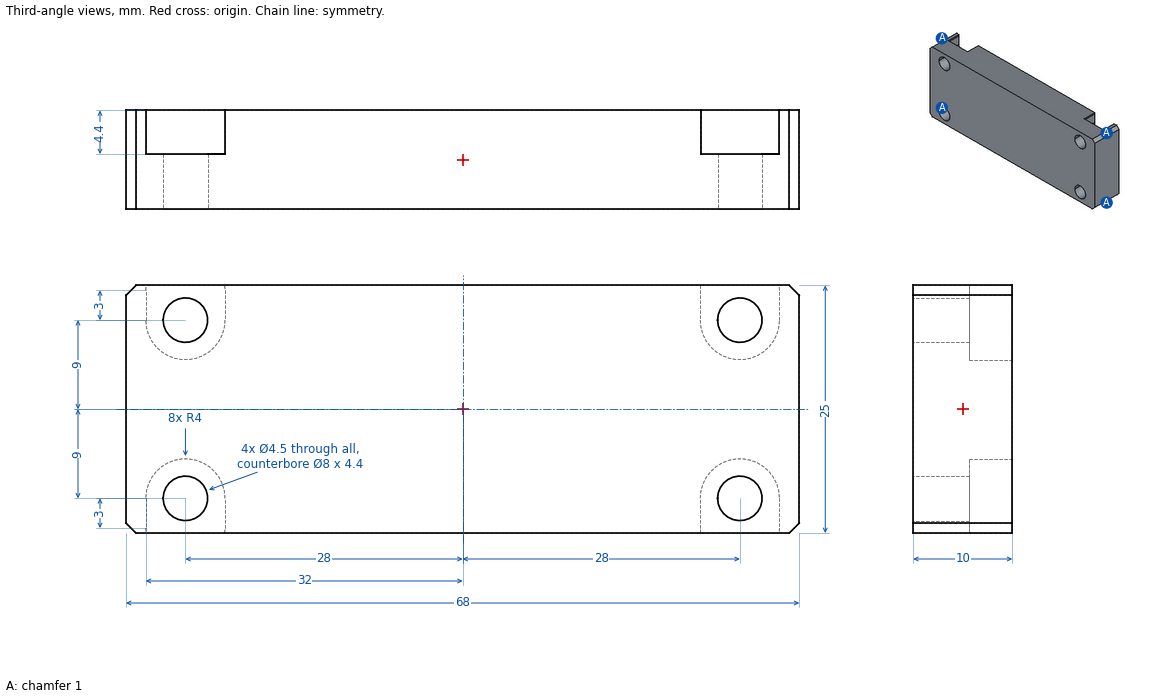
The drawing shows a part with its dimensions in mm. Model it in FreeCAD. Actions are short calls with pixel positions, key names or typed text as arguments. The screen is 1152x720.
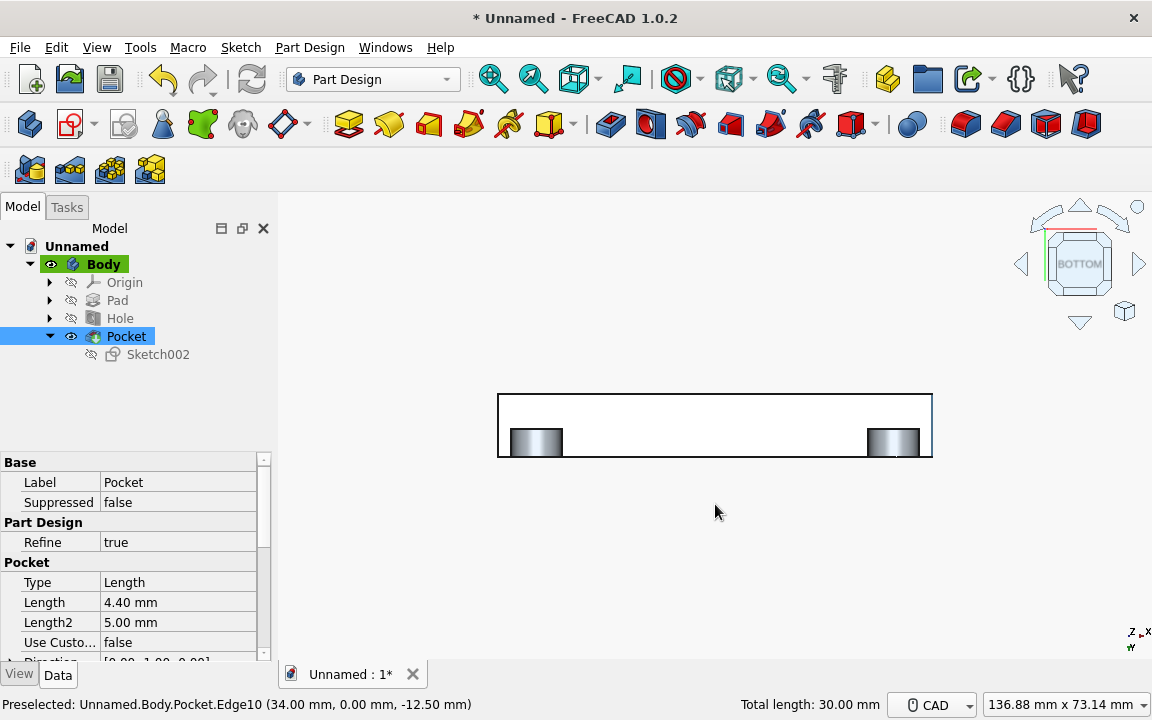
click(498, 424, ctrl)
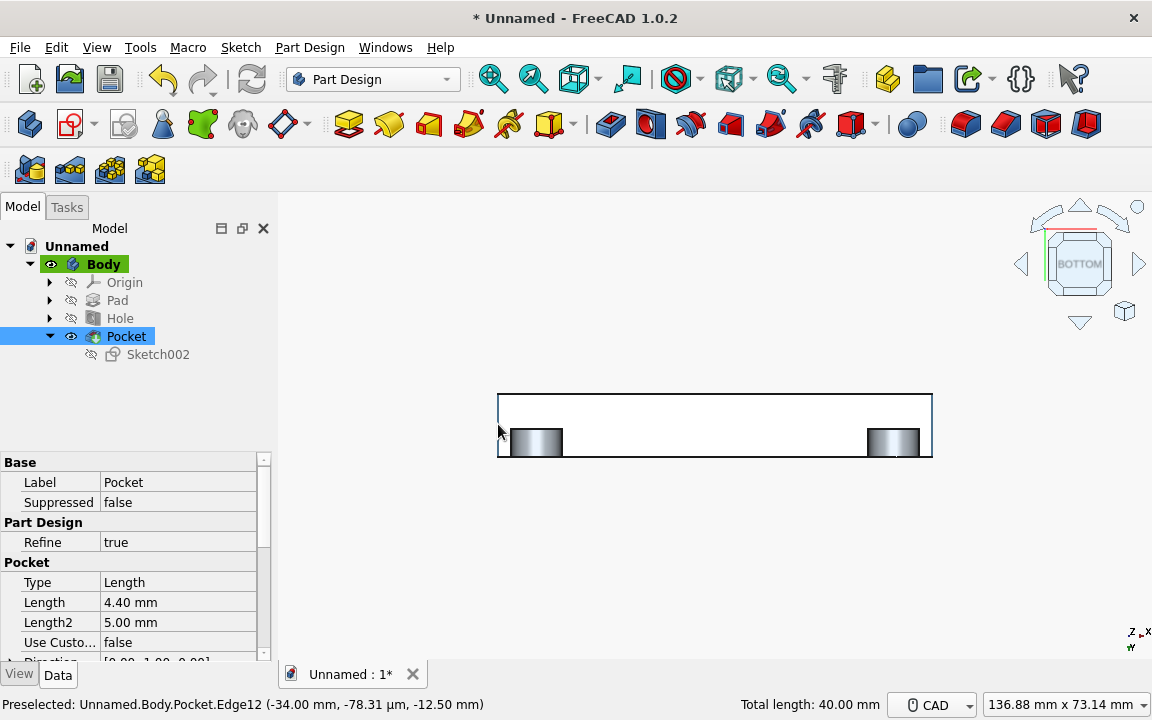
click(1006, 124)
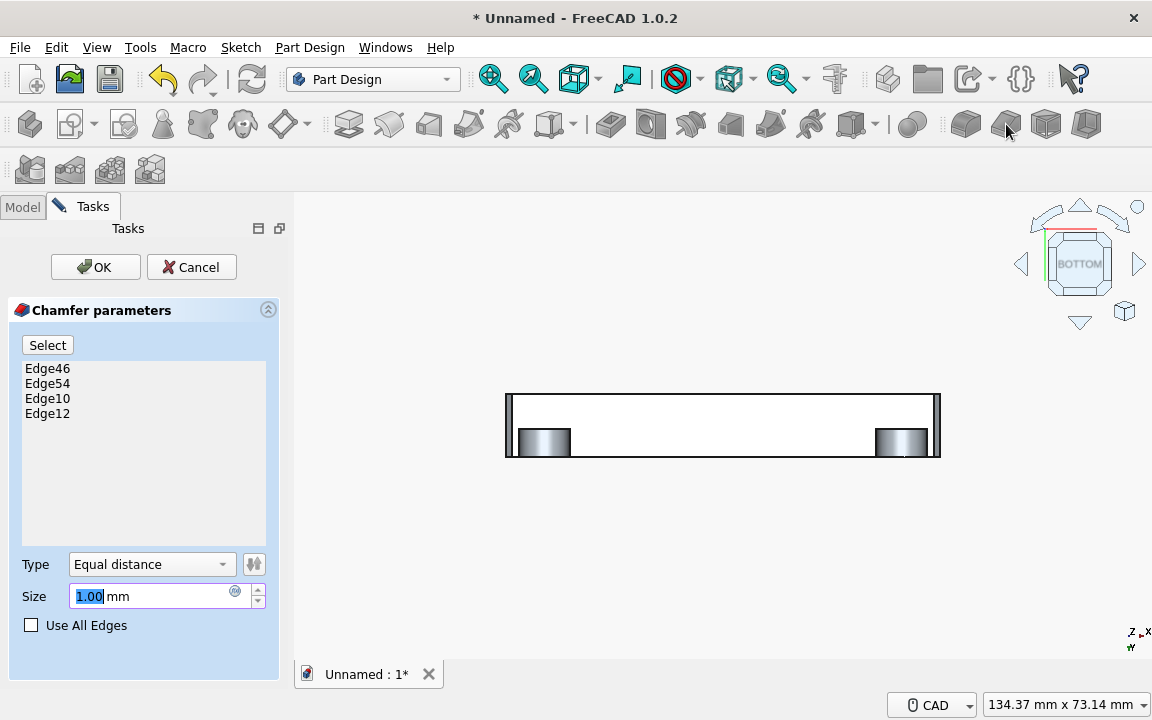
text(1)
key(Tab)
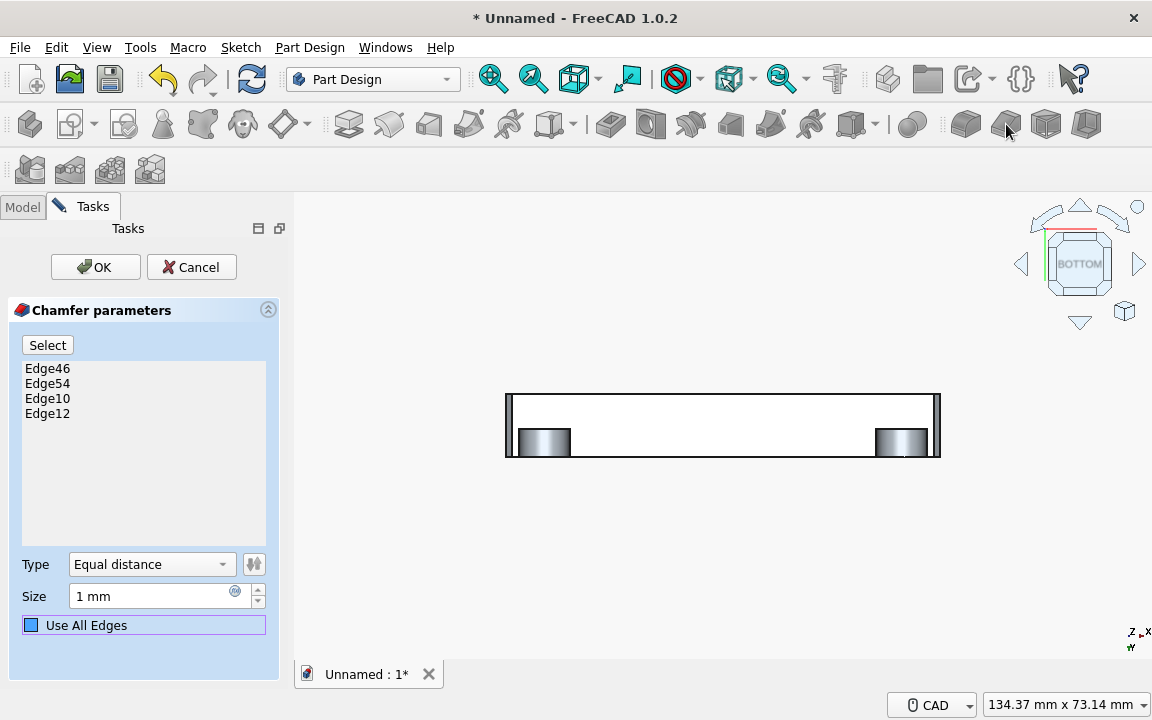
click(96, 267)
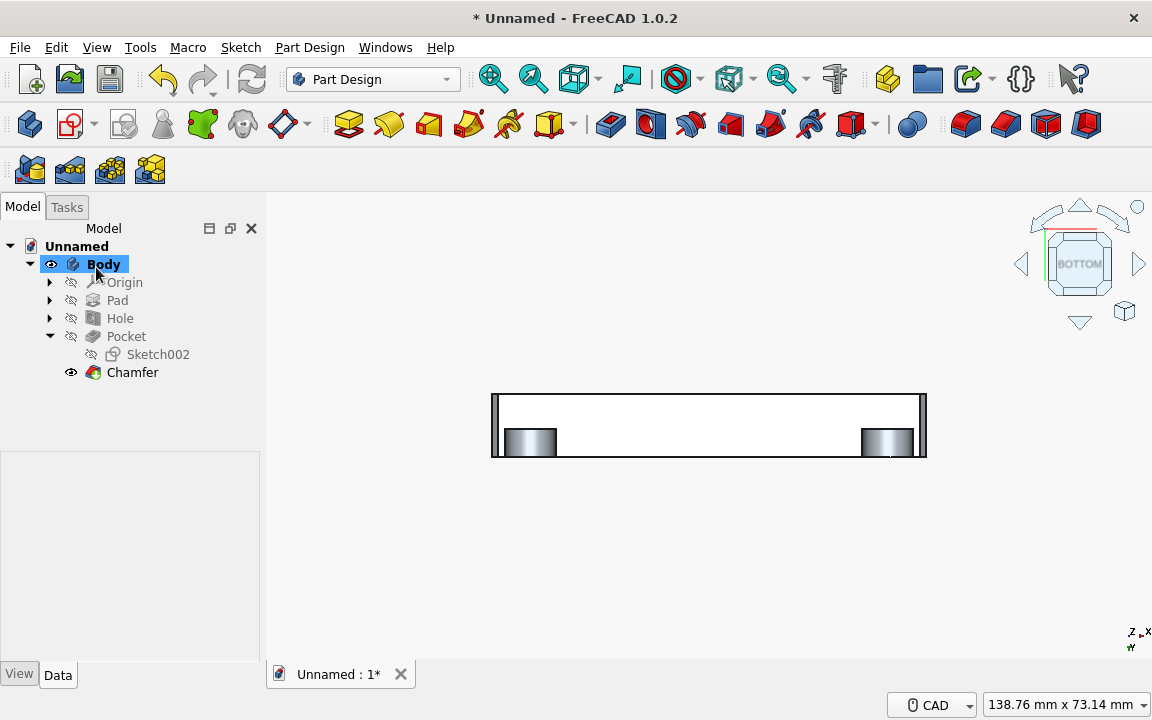
key(0)